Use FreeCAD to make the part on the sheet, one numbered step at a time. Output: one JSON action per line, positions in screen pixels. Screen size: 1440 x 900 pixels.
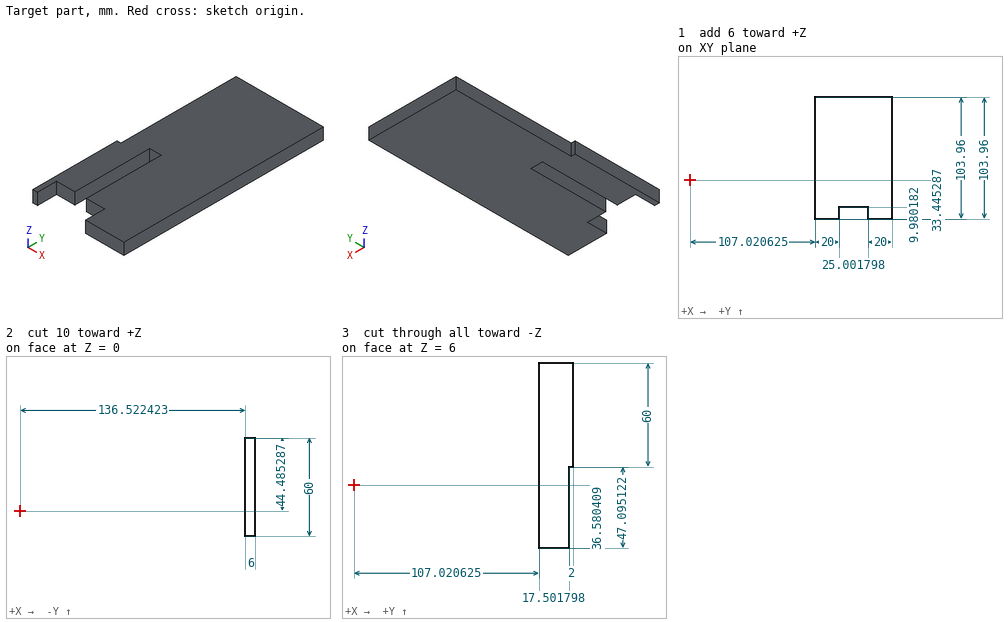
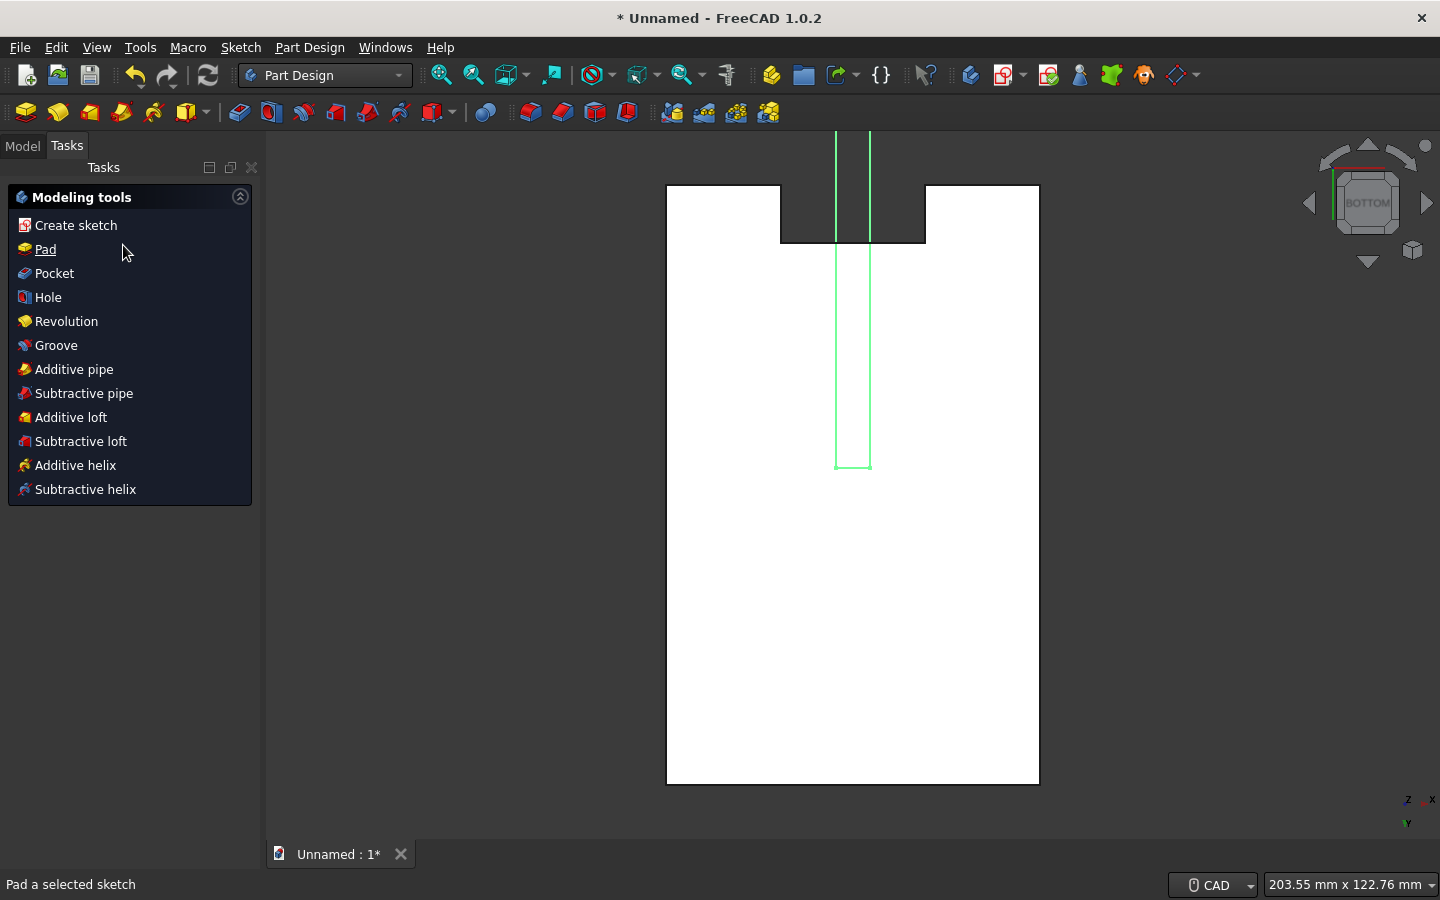
{"action": "left_click", "coordinate": [240, 112]}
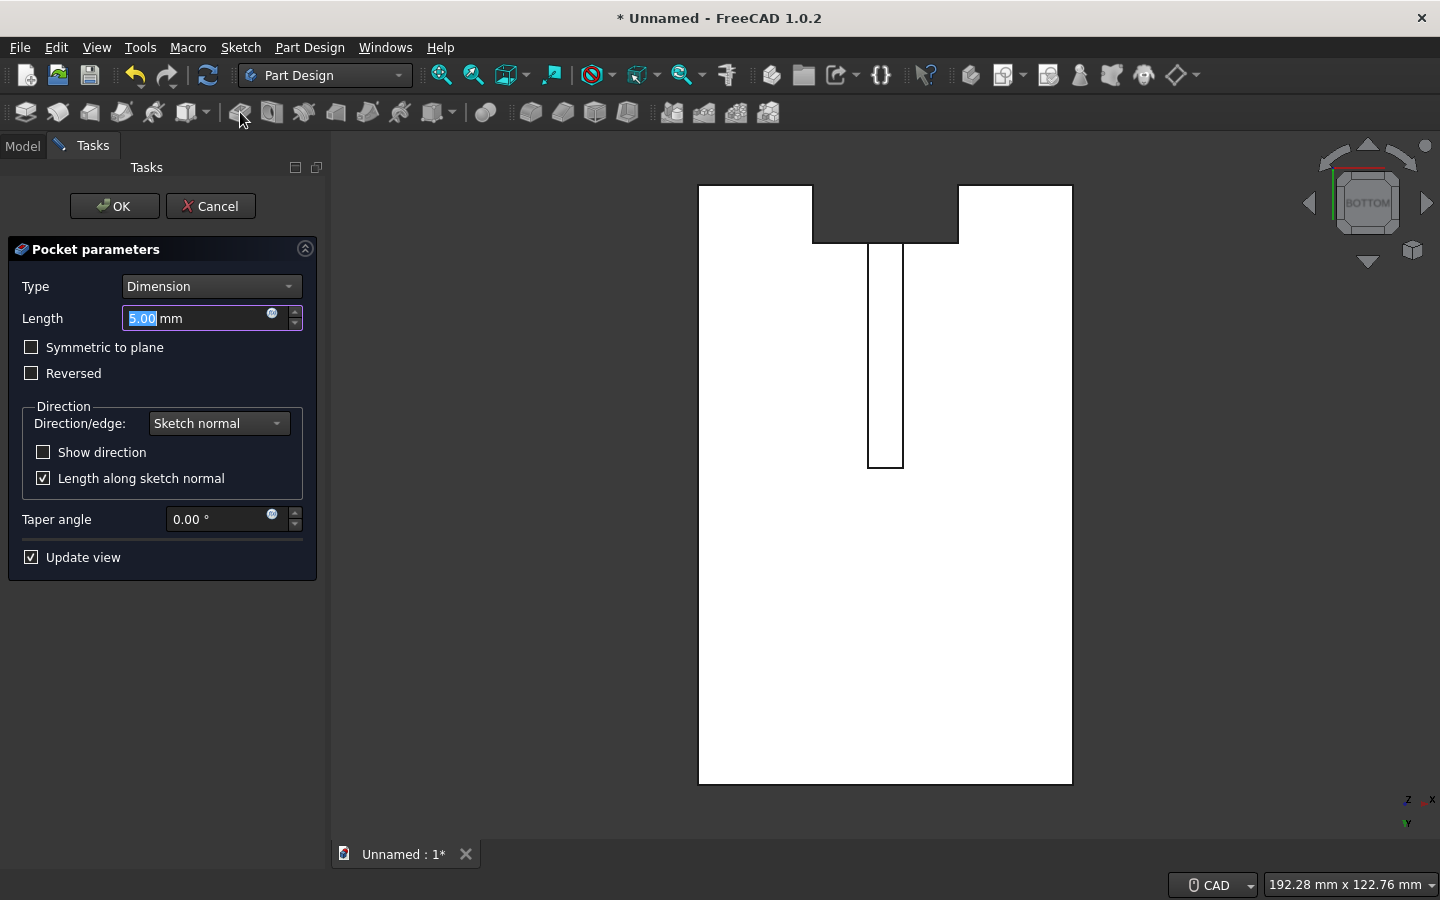
{"action": "type", "text": "10"}
{"action": "key", "text": "Tab"}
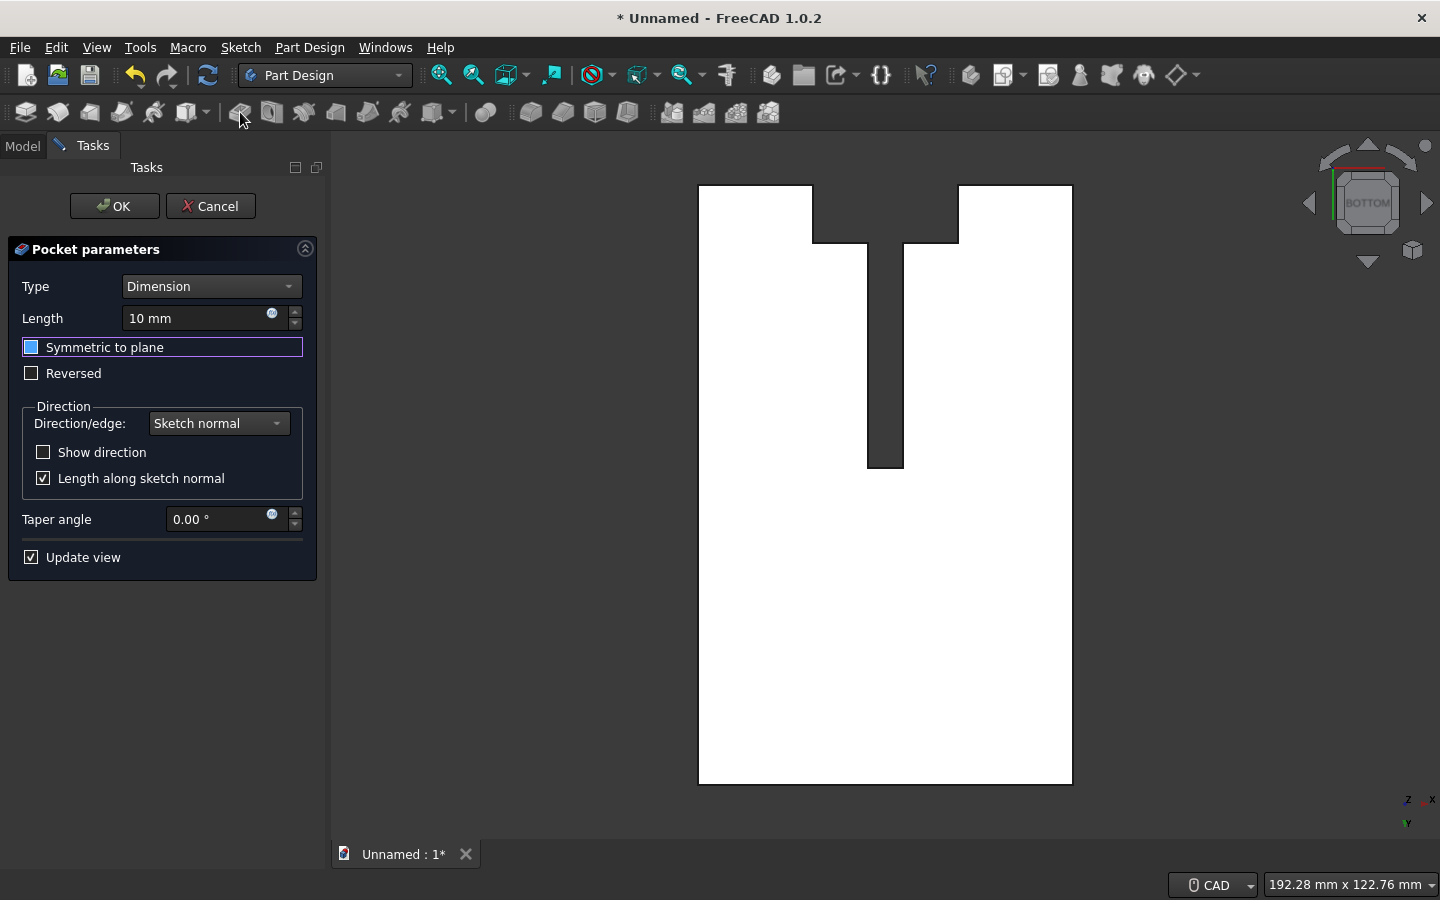
{"action": "left_click", "coordinate": [115, 206]}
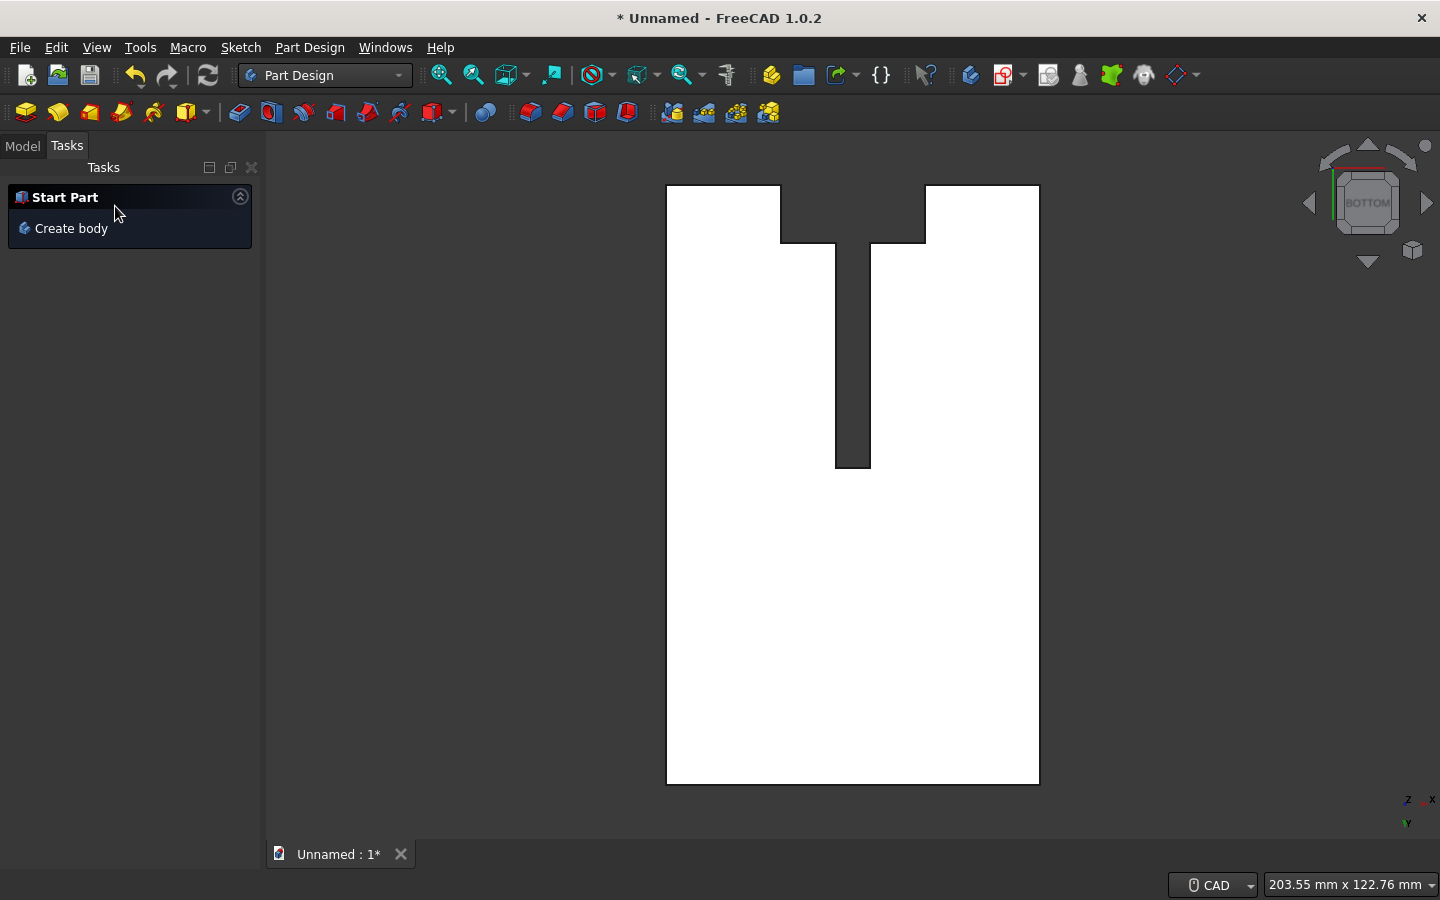
{"action": "key", "text": "0"}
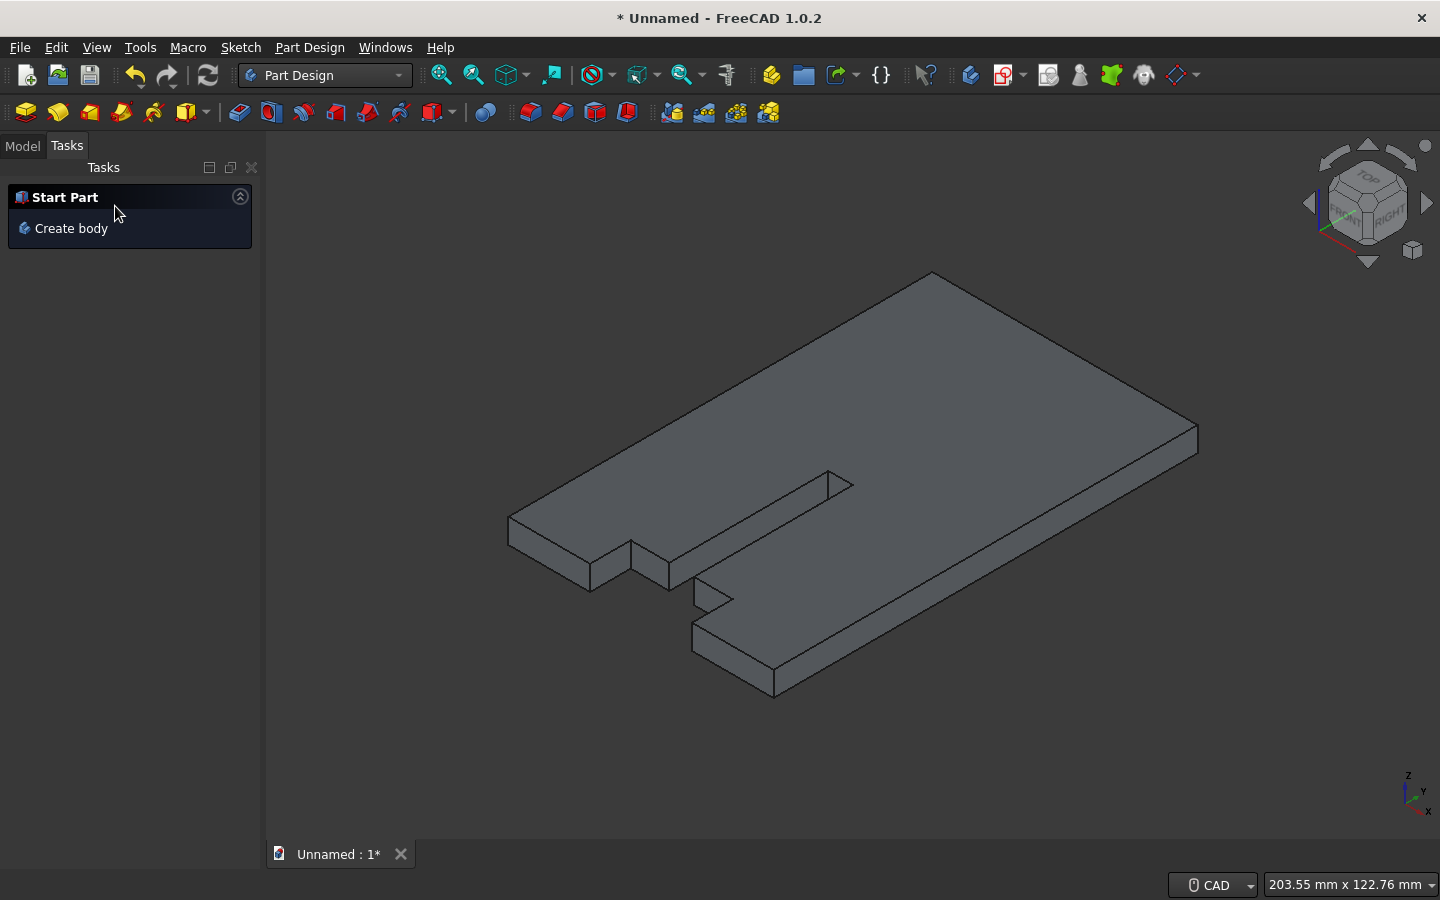
{"action": "left_click", "coordinate": [1012, 422]}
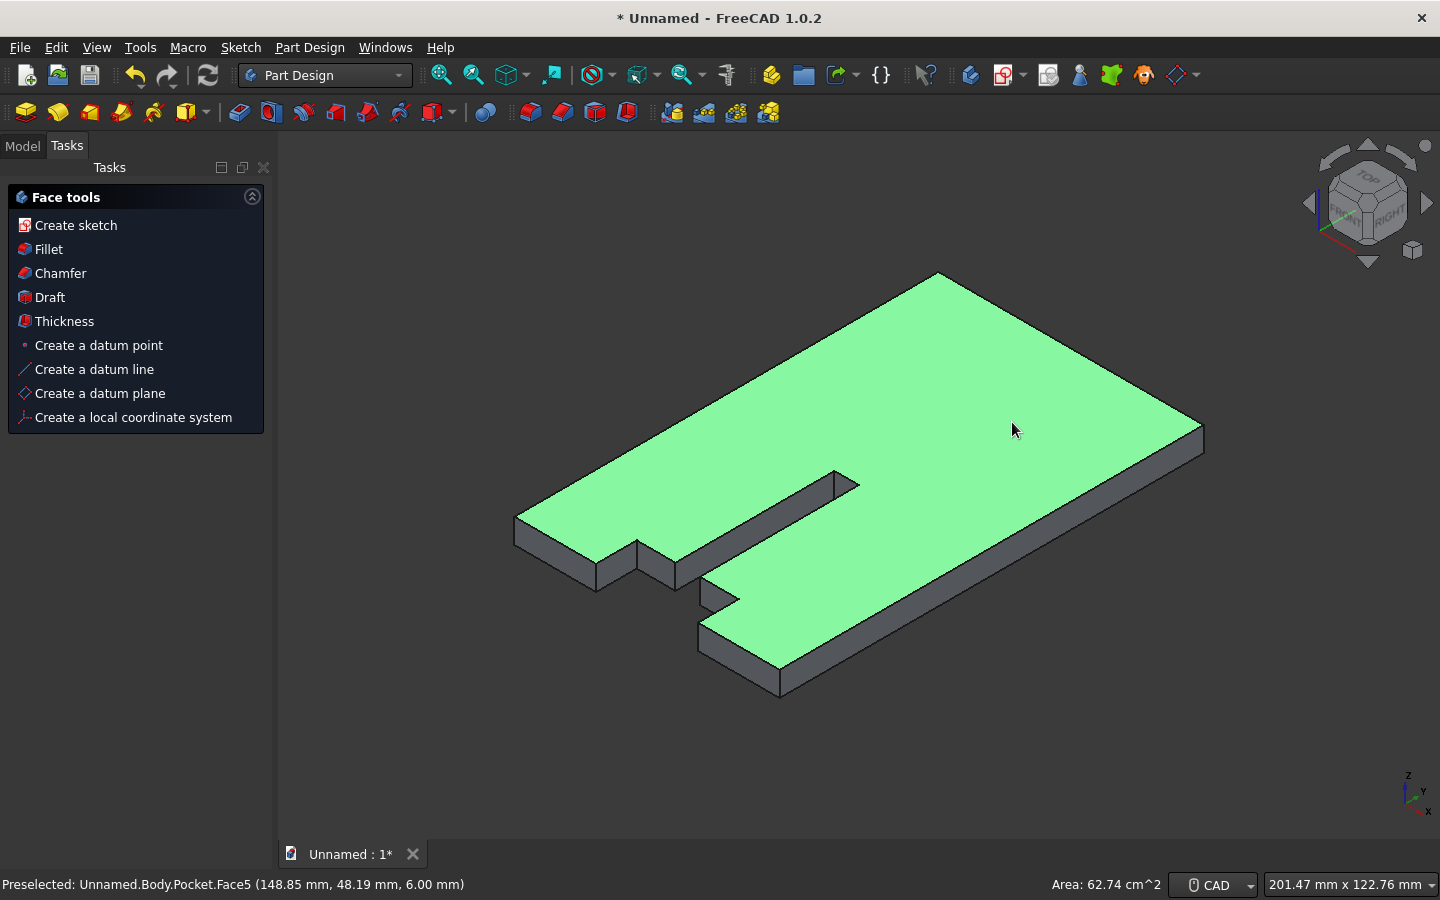
{"action": "left_click", "coordinate": [1004, 76]}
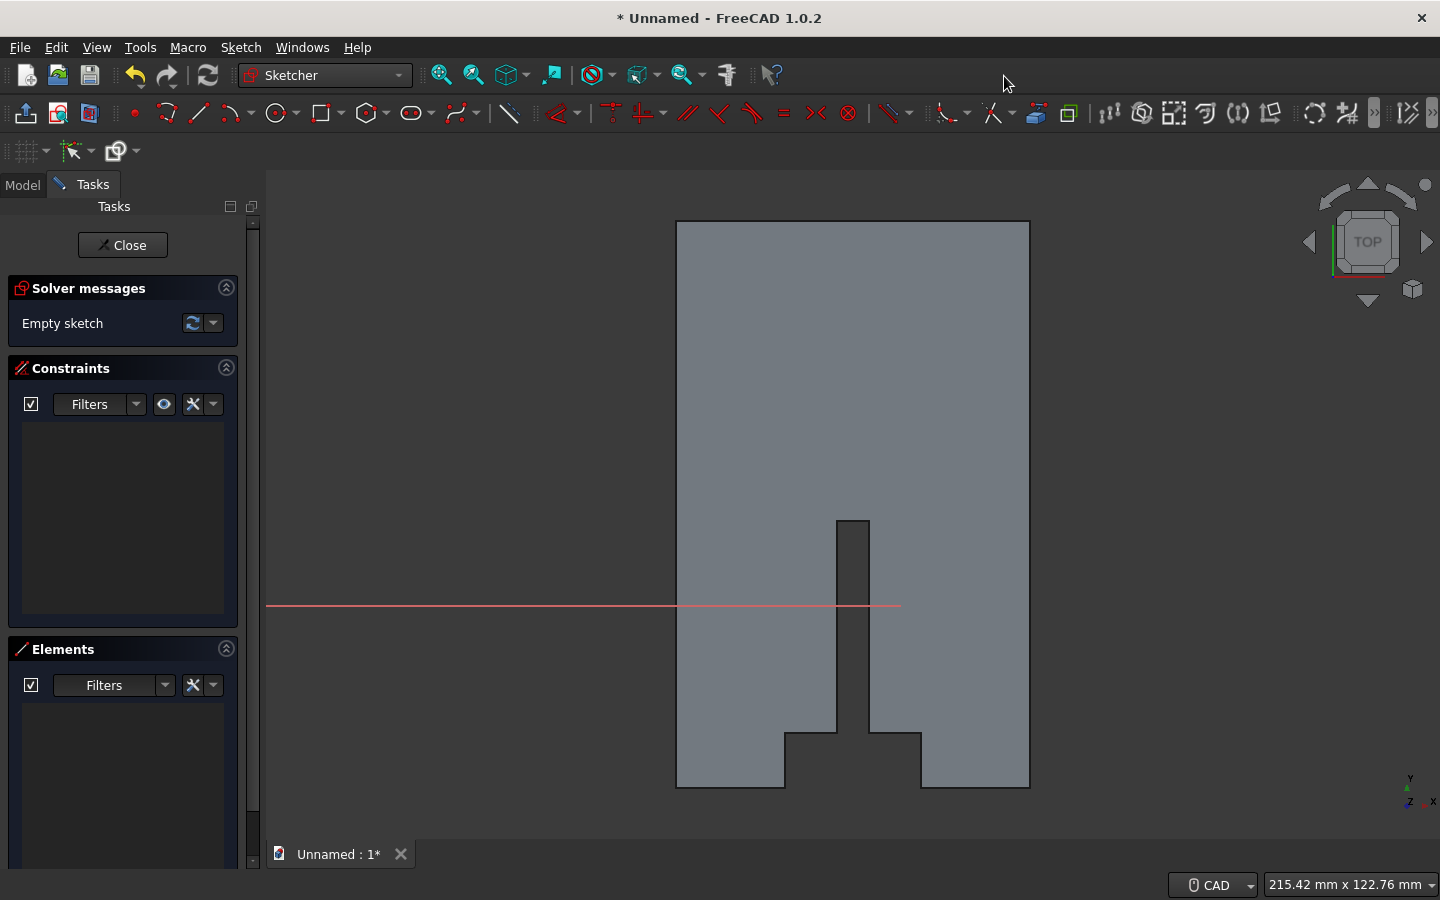
{"action": "scroll", "coordinate": [1275, 487], "scroll_direction": "down", "scroll_amount": 2}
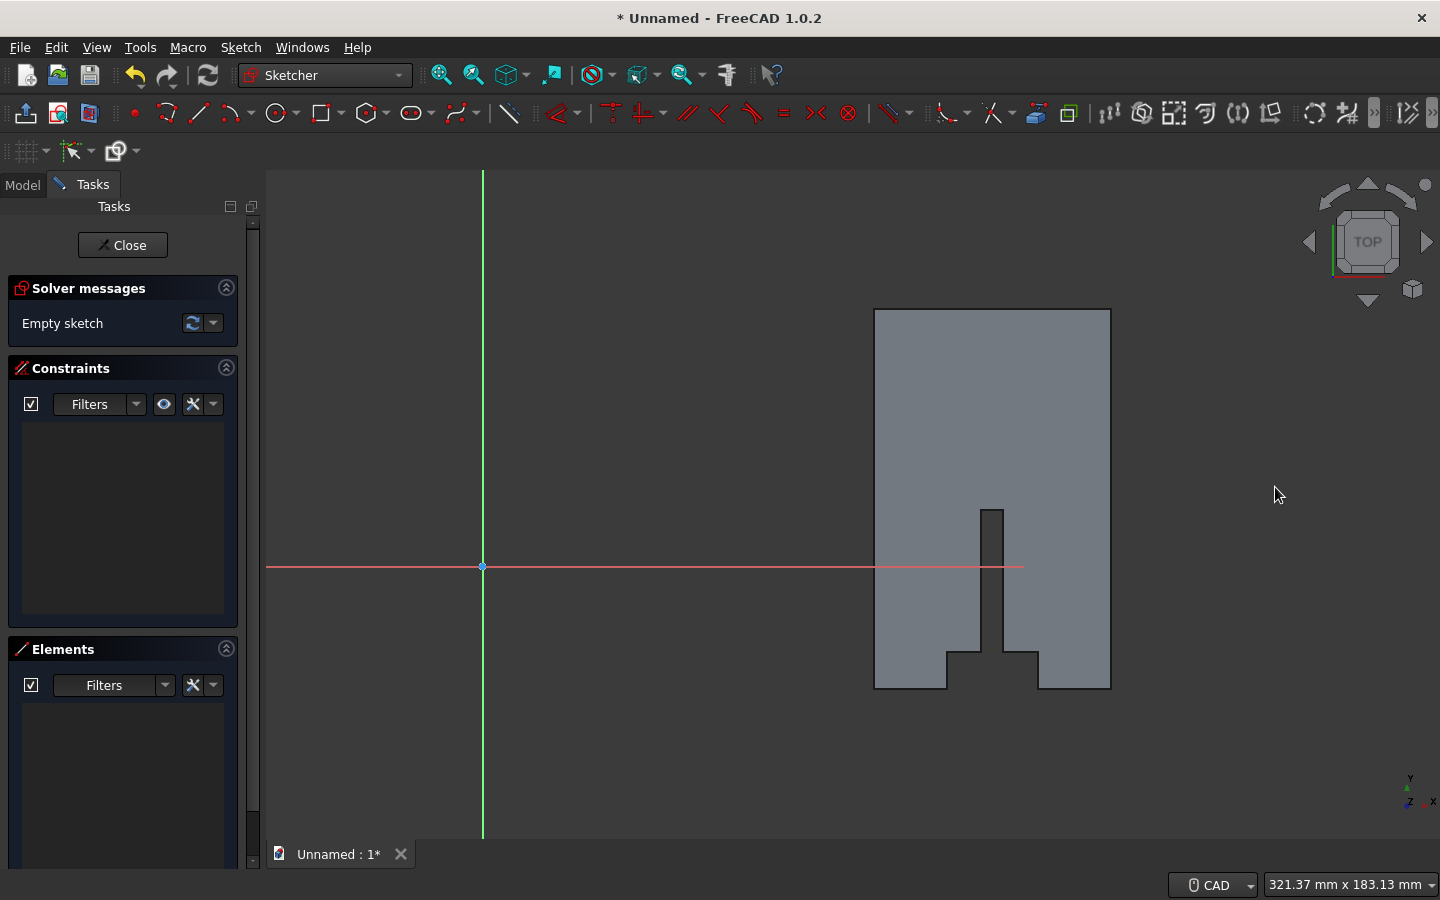
{"action": "left_click", "coordinate": [168, 114]}